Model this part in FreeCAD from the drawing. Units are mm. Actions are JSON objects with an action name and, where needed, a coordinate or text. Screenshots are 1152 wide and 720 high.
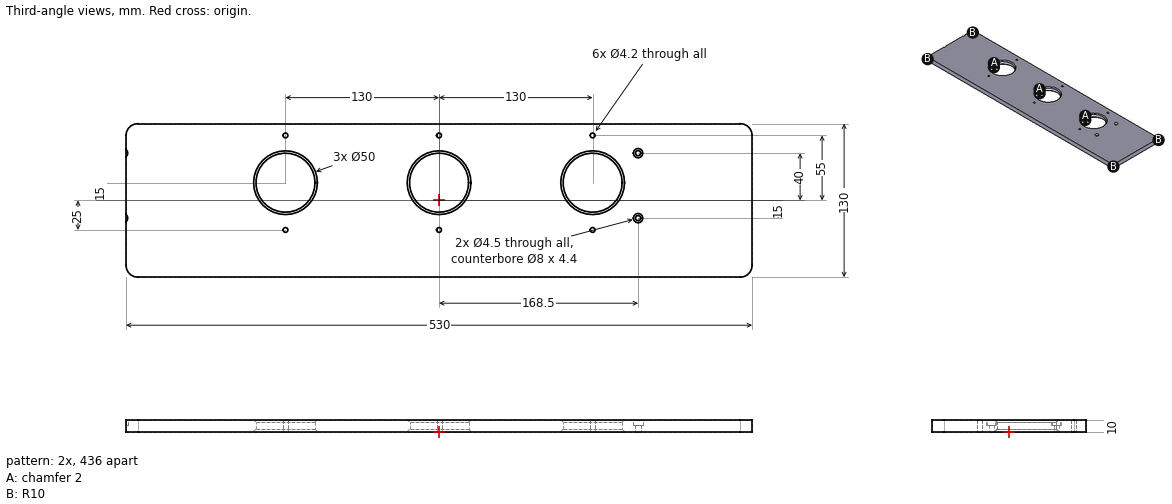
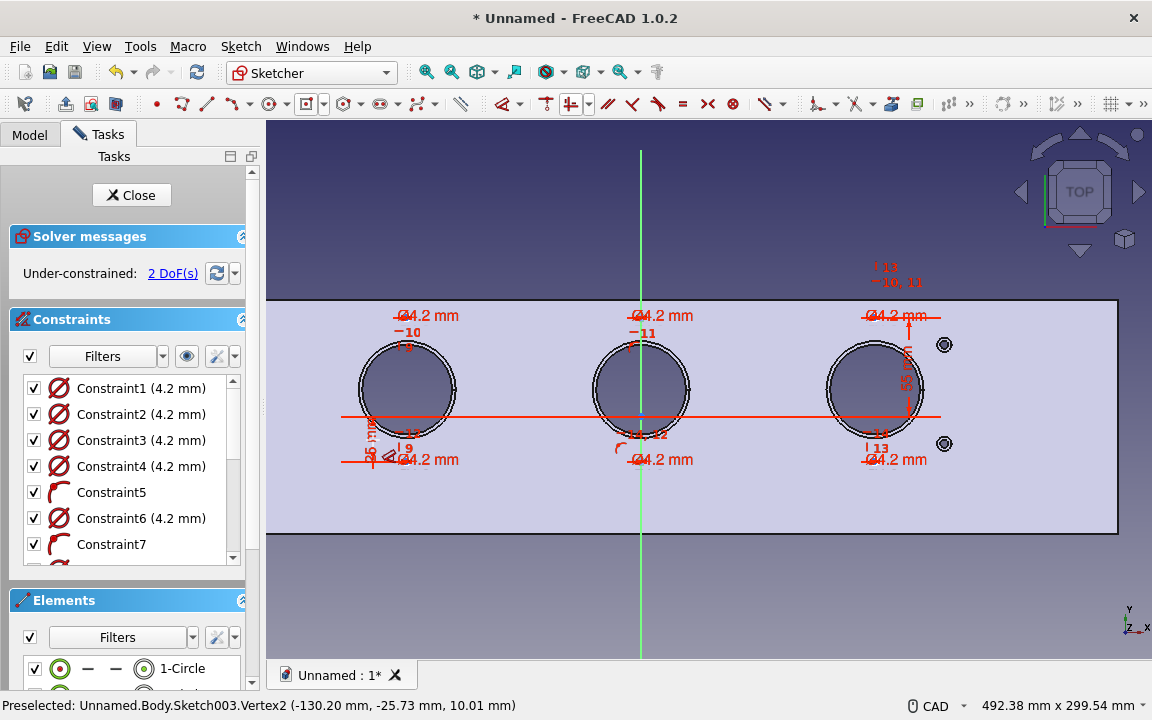
{"action": "left_click", "coordinate": [875, 318]}
{"action": "left_click", "coordinate": [758, 284]}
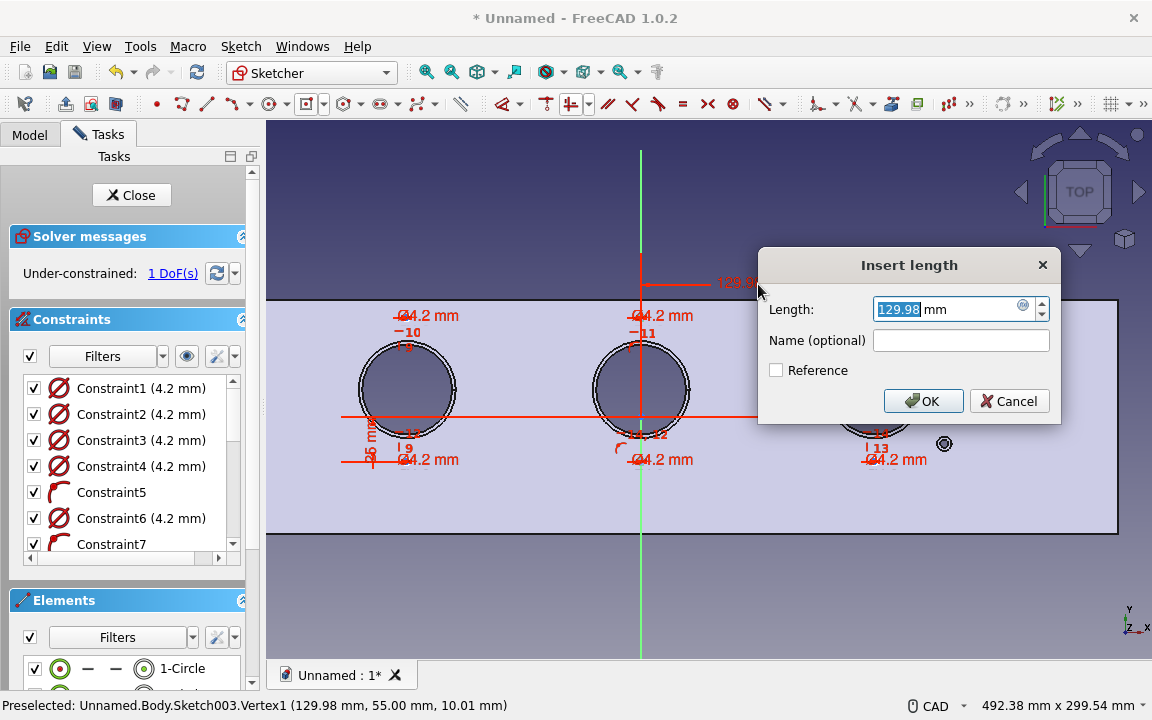
{"action": "type", "text": "130"}
{"action": "key", "text": "Return"}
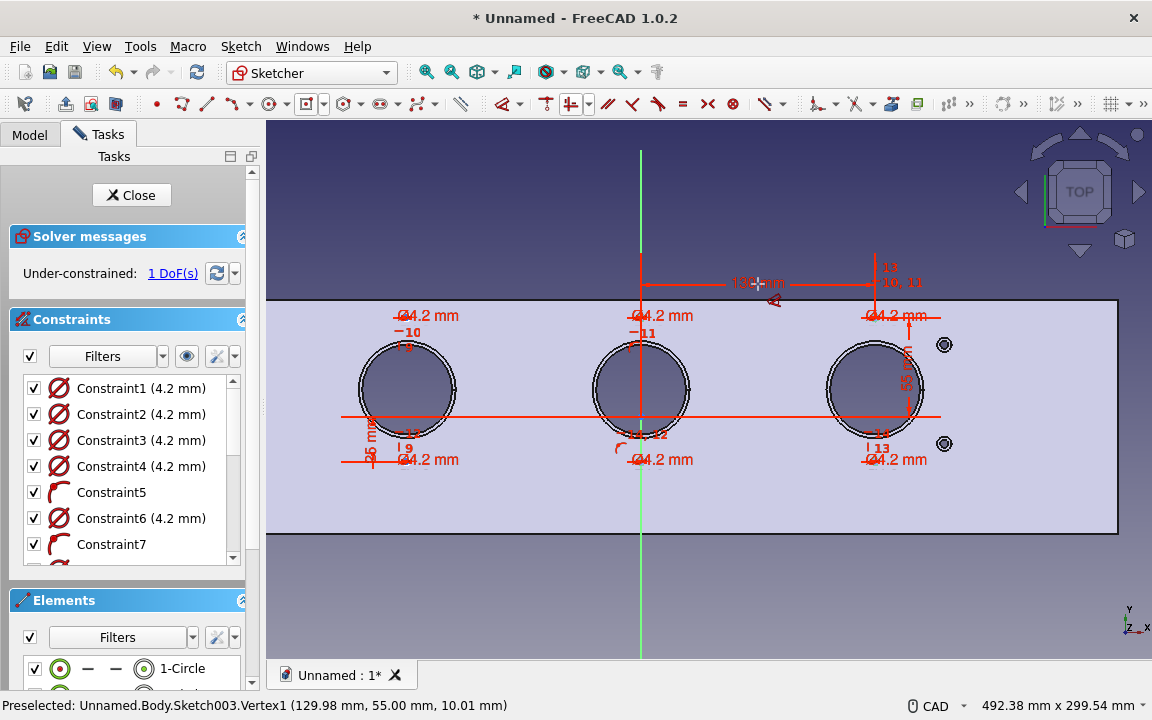
{"action": "left_click", "coordinate": [407, 462]}
{"action": "left_click", "coordinate": [524, 496]}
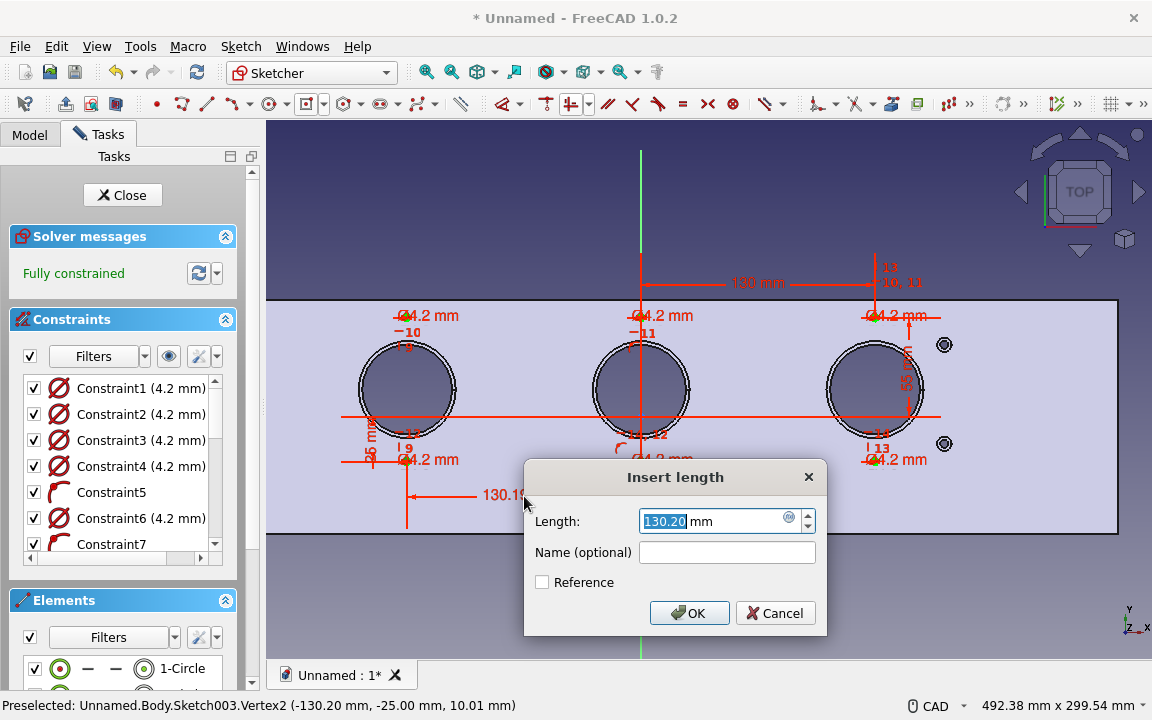
{"action": "type", "text": "130"}
{"action": "key", "text": "Return"}
{"action": "key", "text": "Escape"}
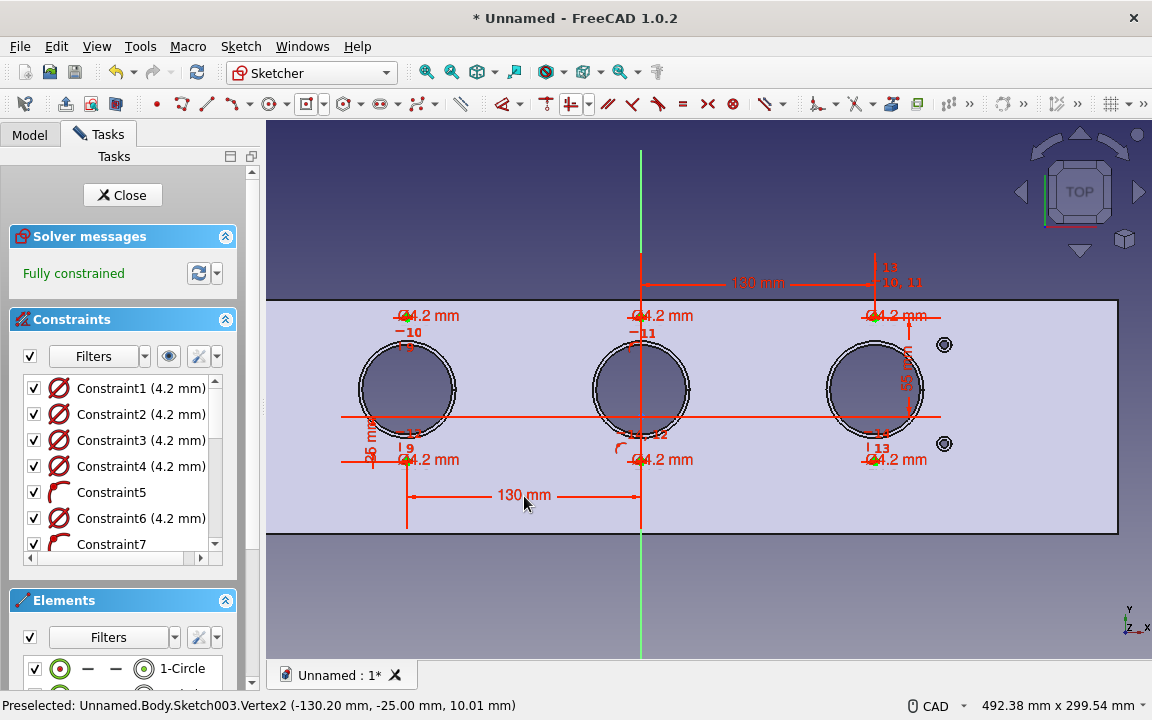
{"action": "left_click", "coordinate": [123, 195]}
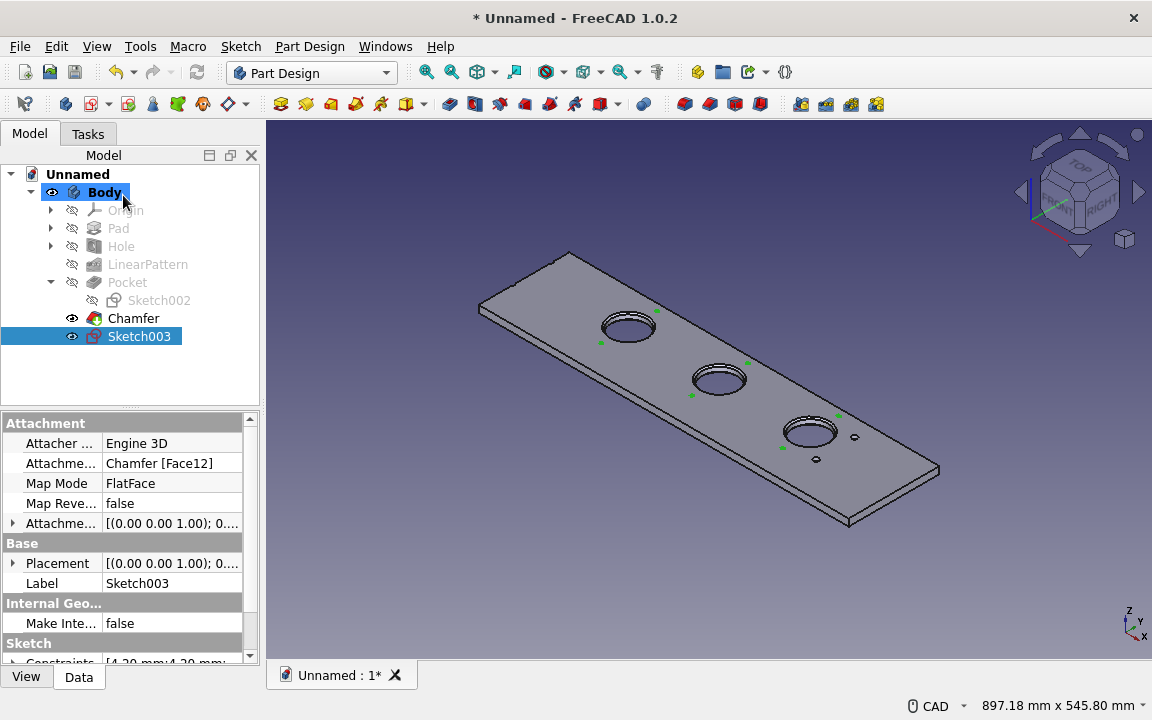
{"action": "left_click", "coordinate": [475, 104]}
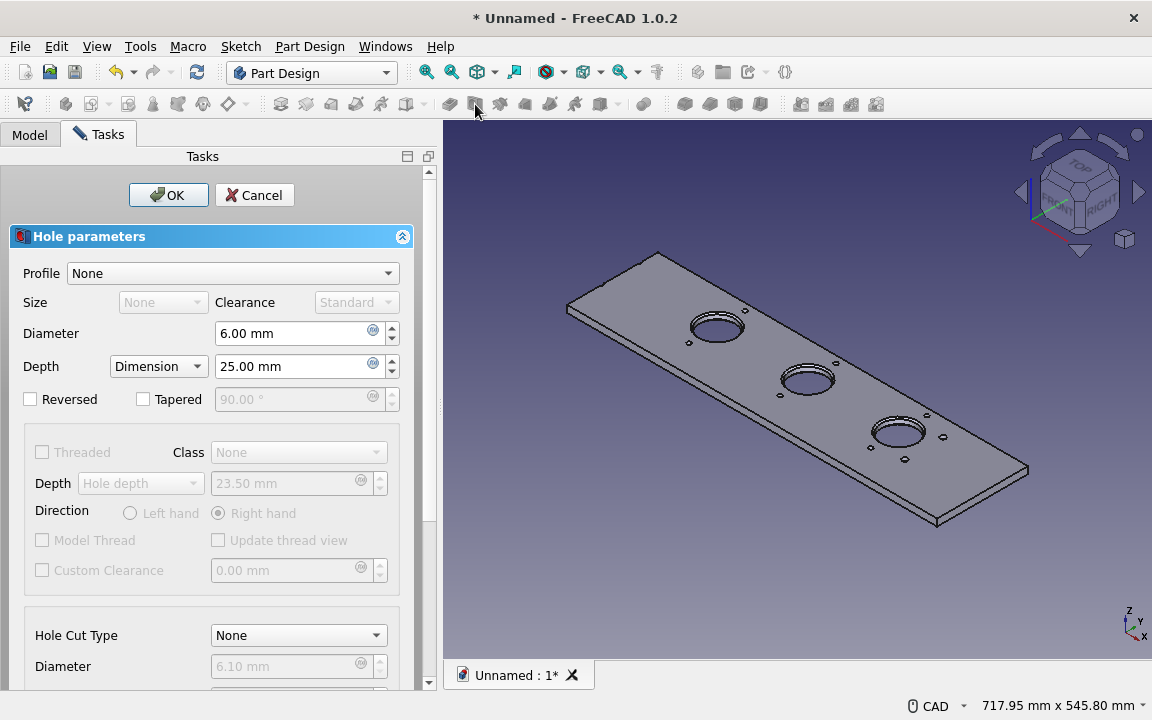
{"action": "triple_click", "coordinate": [300, 334]}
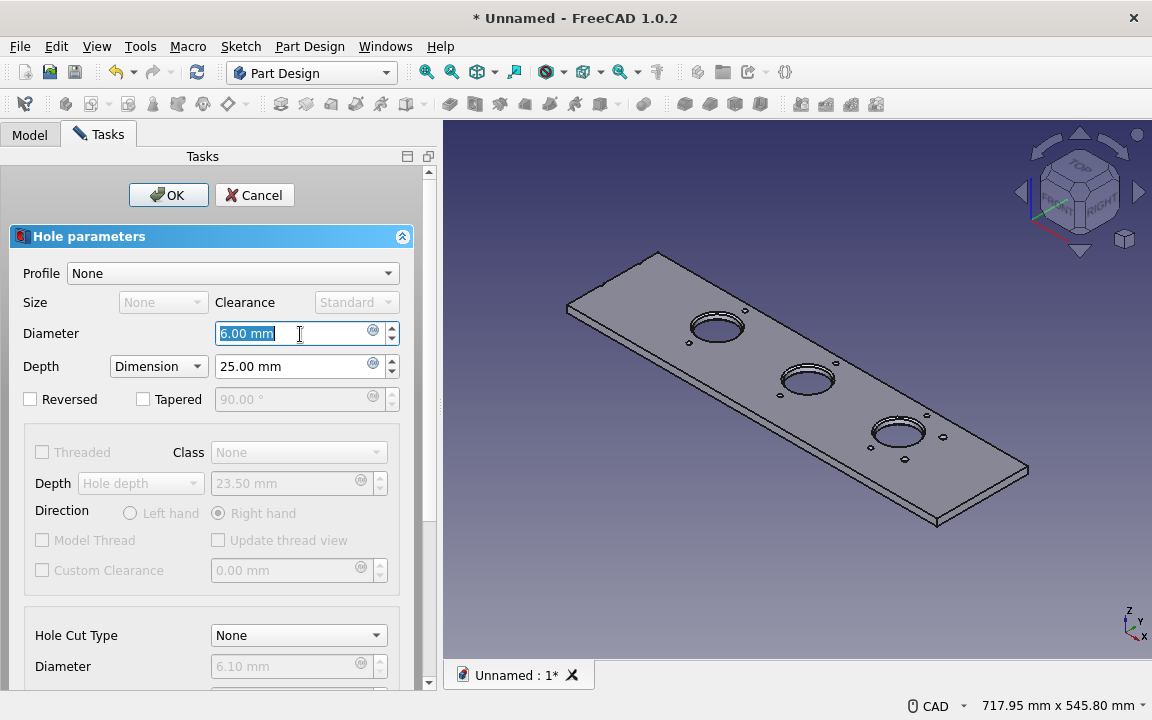
{"action": "type", "text": "4.2"}
{"action": "key", "text": "Tab"}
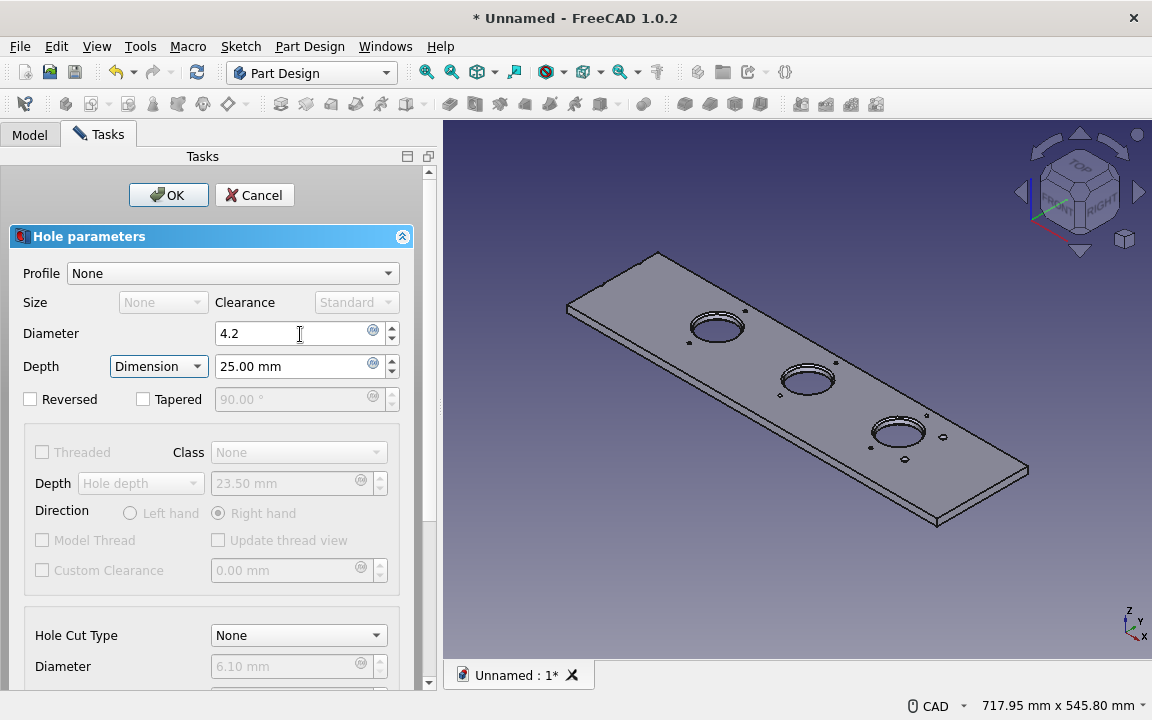
{"action": "left_click", "coordinate": [160, 366]}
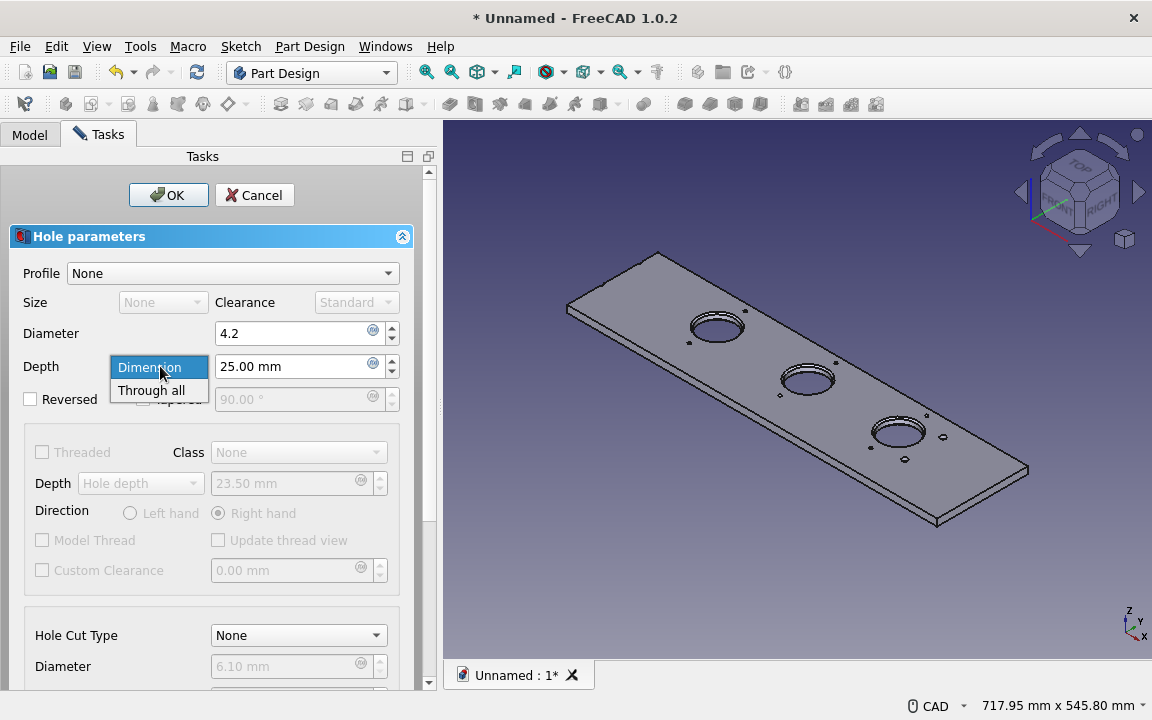
{"action": "left_click", "coordinate": [158, 390]}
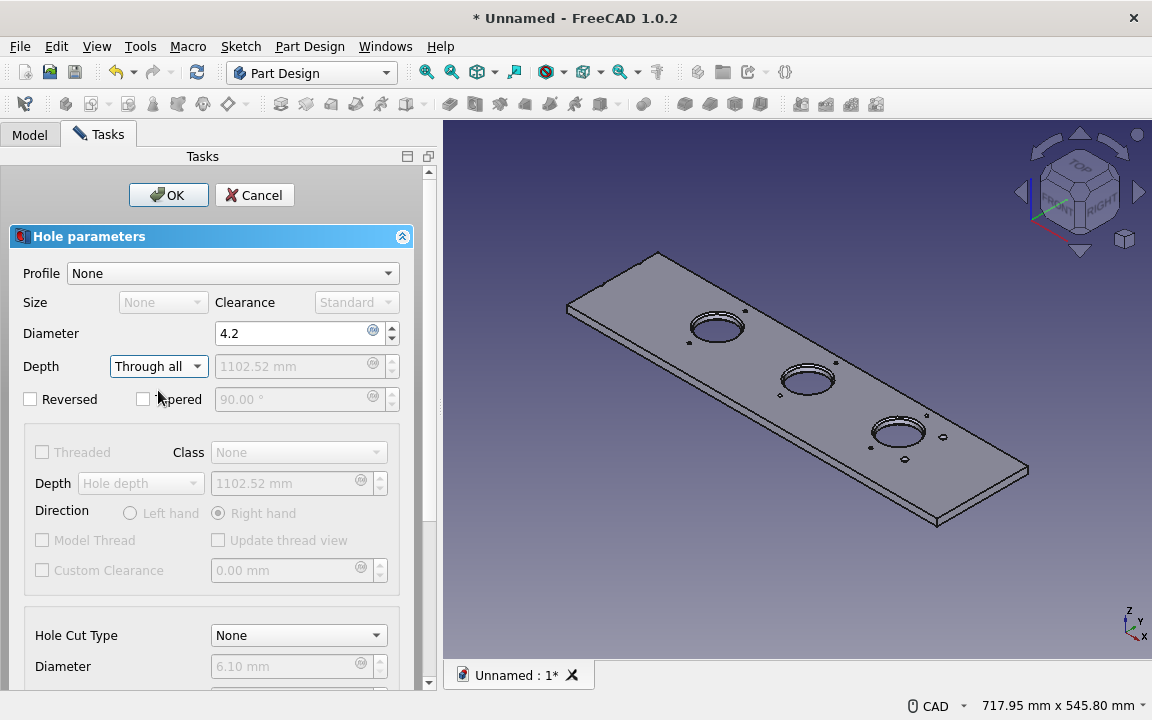
{"action": "left_click", "coordinate": [169, 195]}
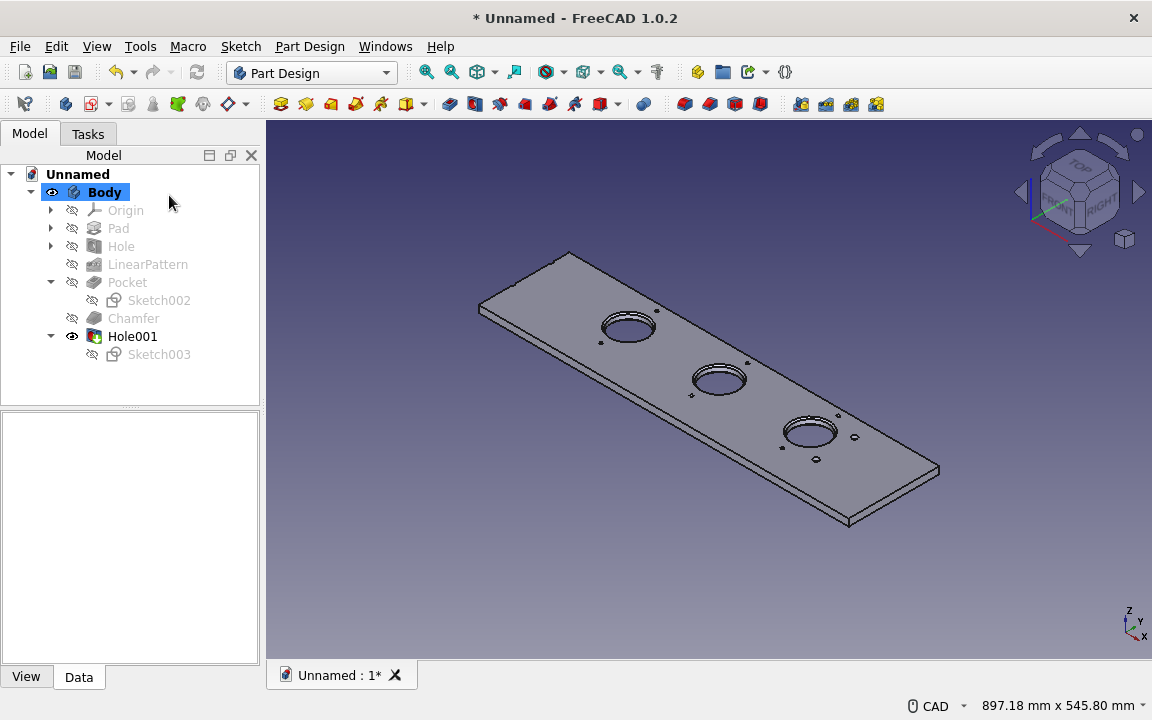
{"action": "left_click", "coordinate": [849, 524]}